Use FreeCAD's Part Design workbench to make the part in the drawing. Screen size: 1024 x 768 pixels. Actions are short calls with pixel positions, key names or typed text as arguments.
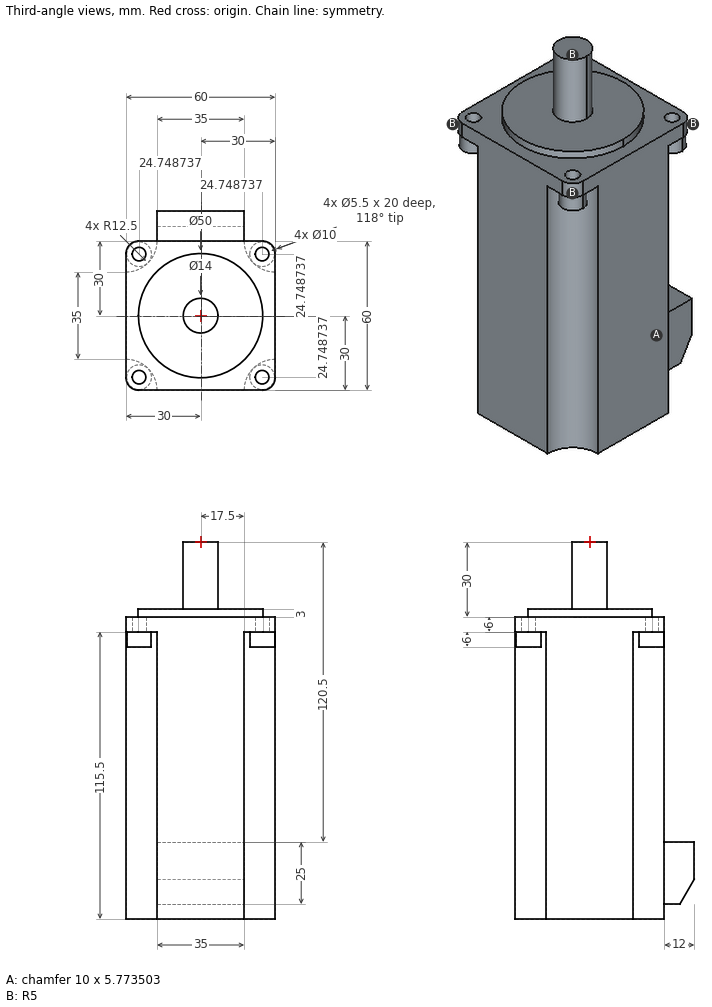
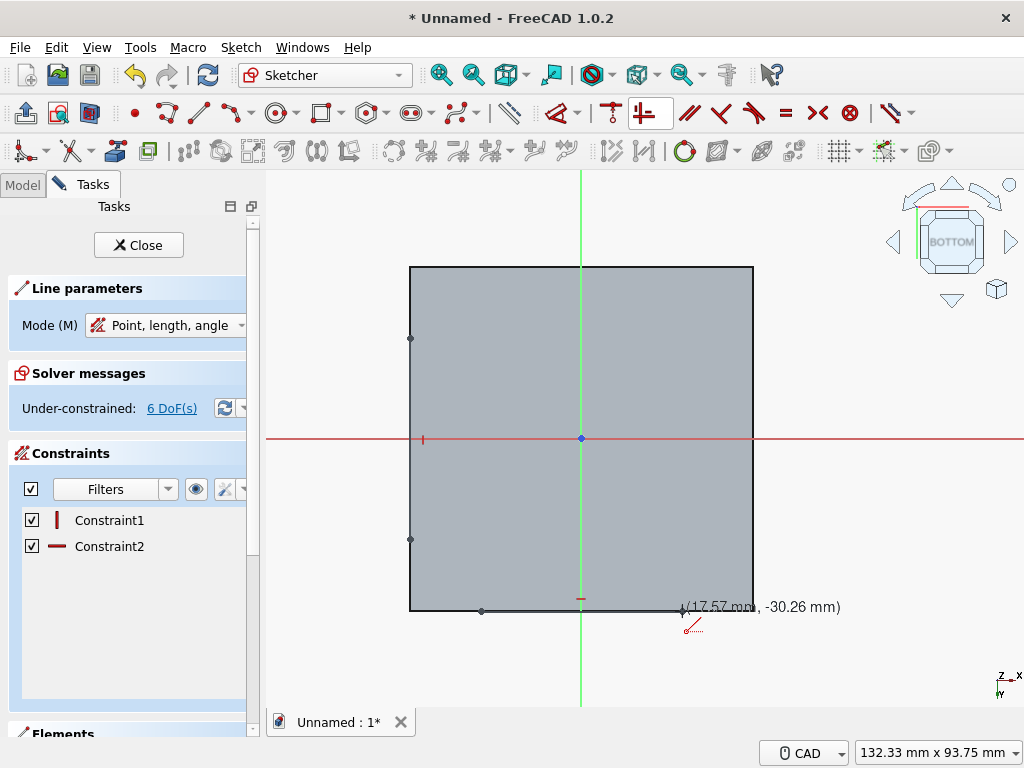
click(753, 539)
click(753, 338)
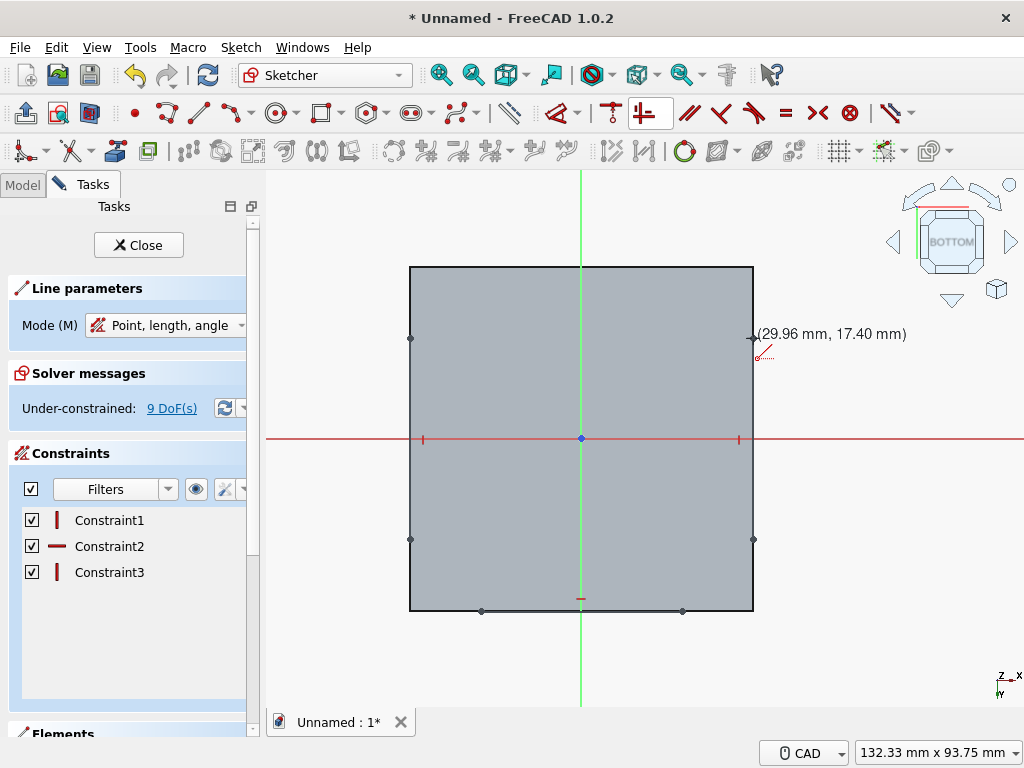
click(682, 267)
click(481, 267)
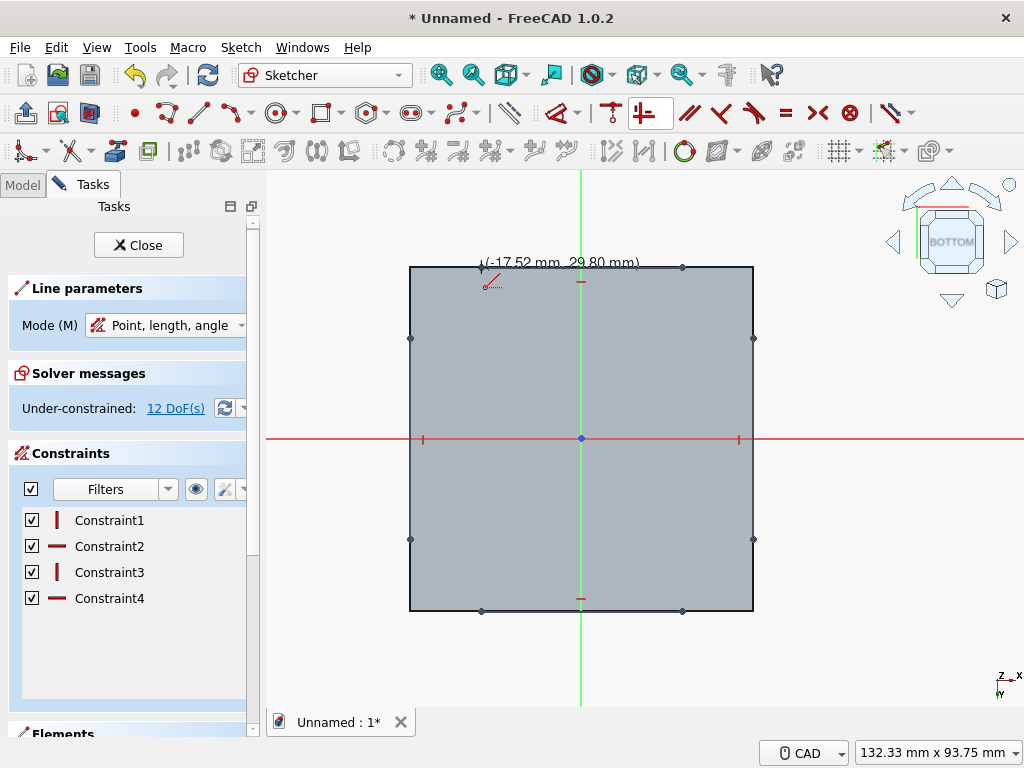
click(232, 114)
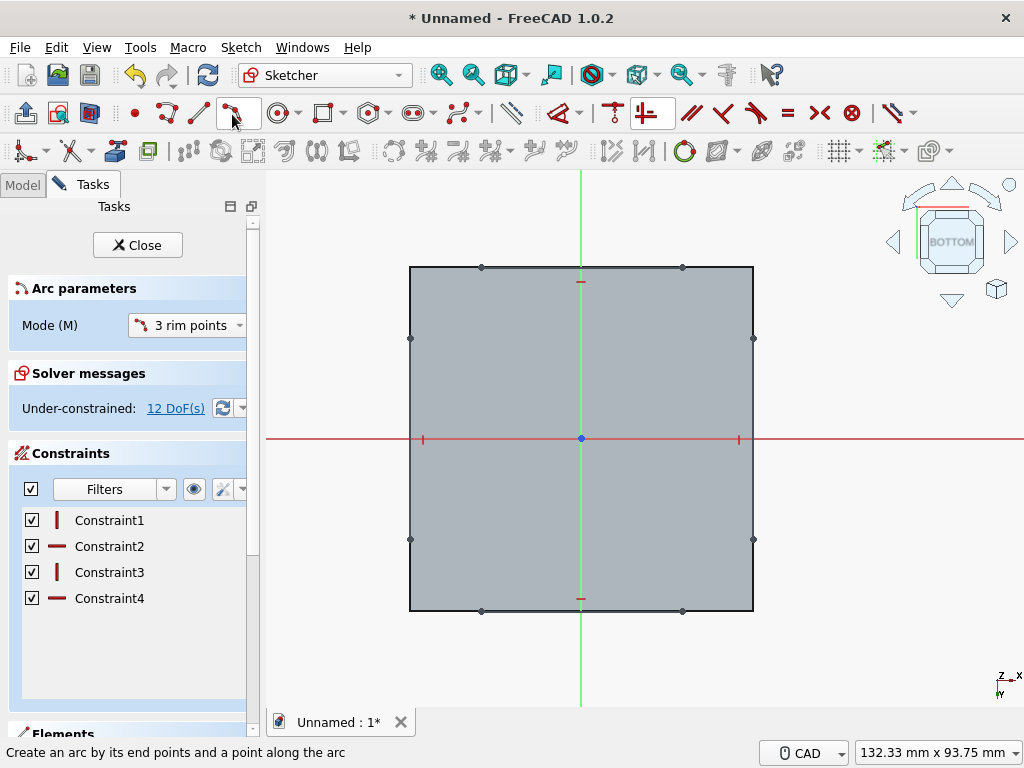
click(410, 540)
click(481, 612)
click(460, 560)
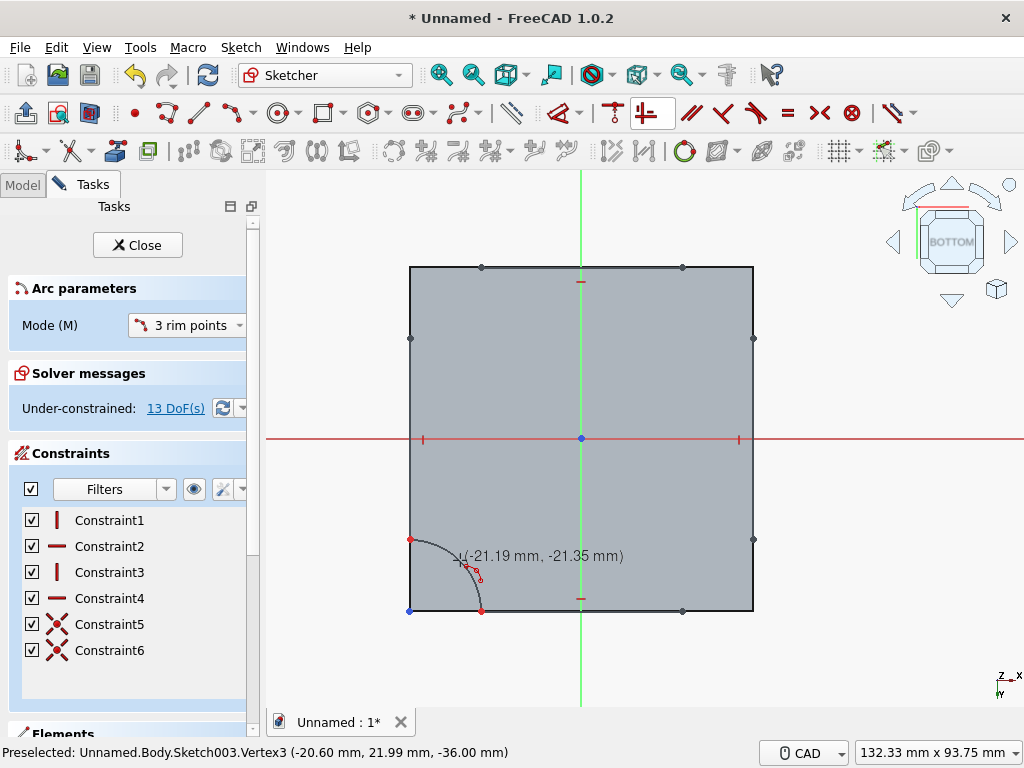
click(682, 612)
click(753, 540)
click(703, 560)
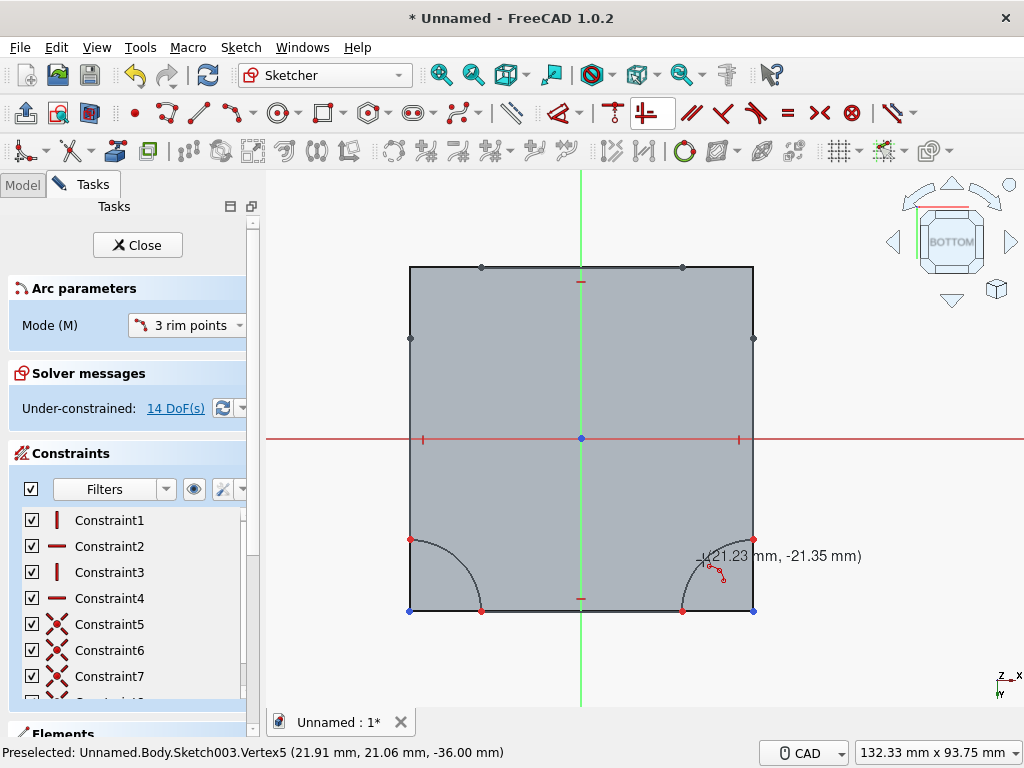
click(753, 339)
click(682, 268)
click(703, 317)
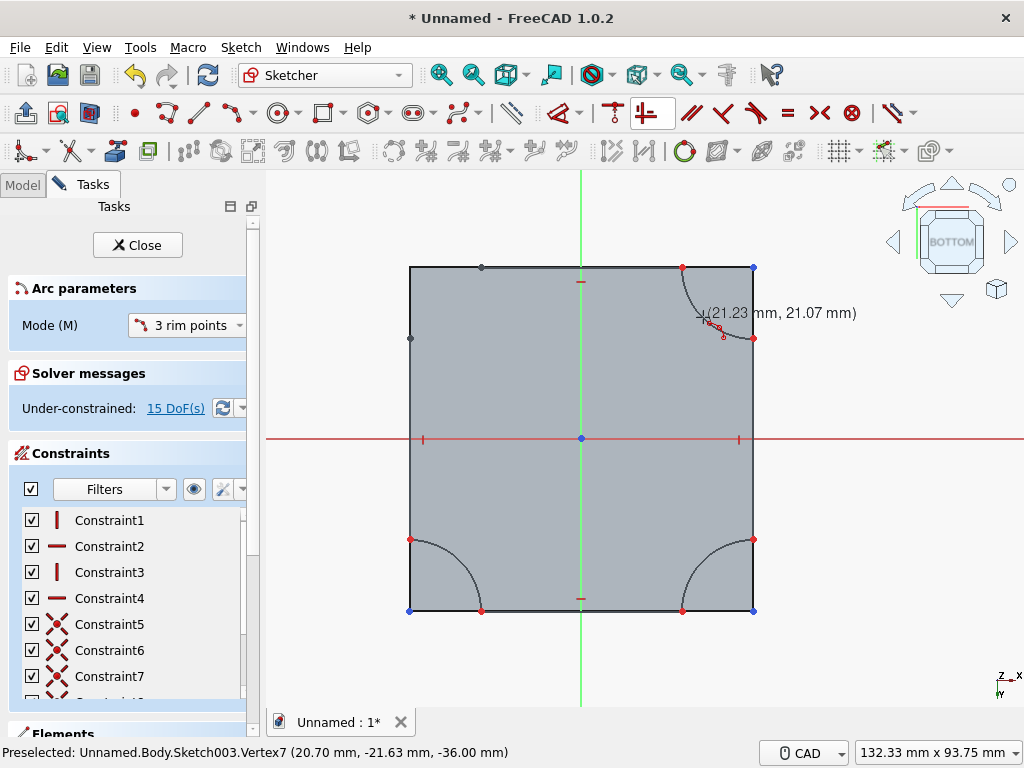
click(481, 268)
click(410, 339)
click(460, 317)
key(Escape)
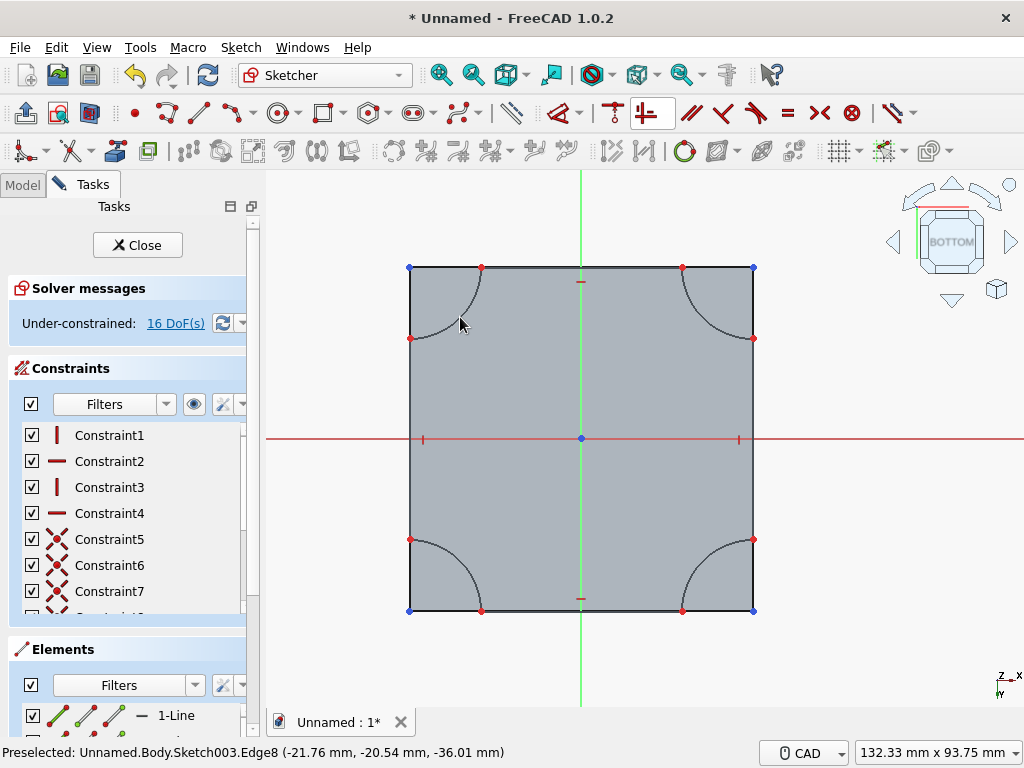
click(473, 580)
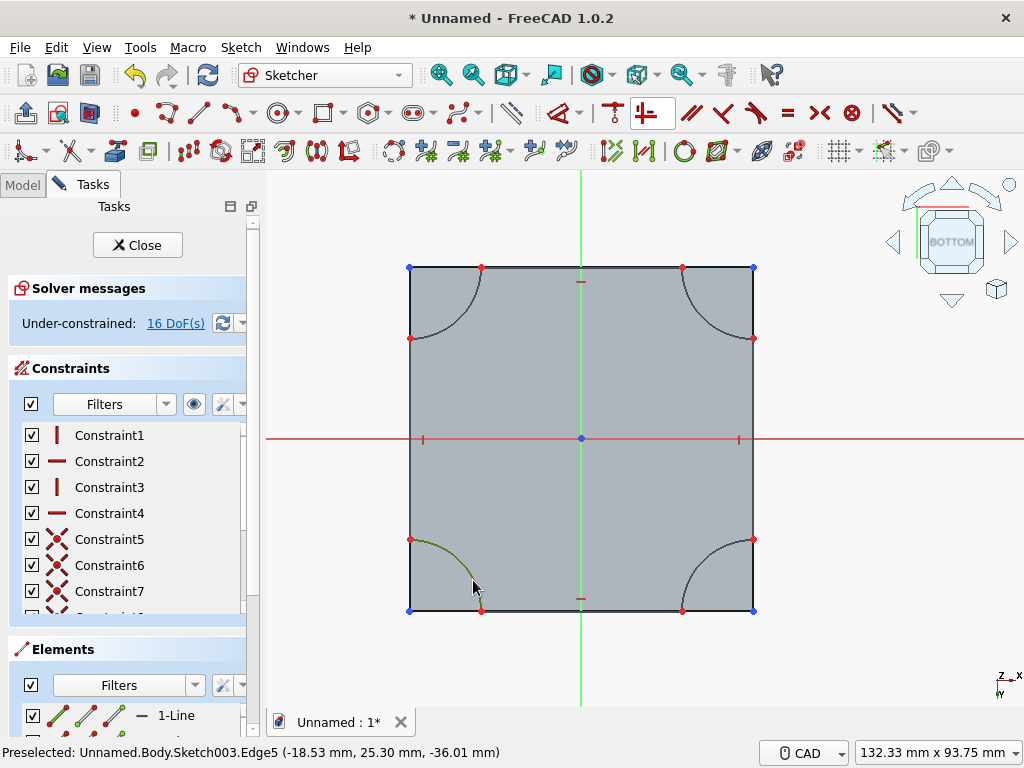
click(721, 548)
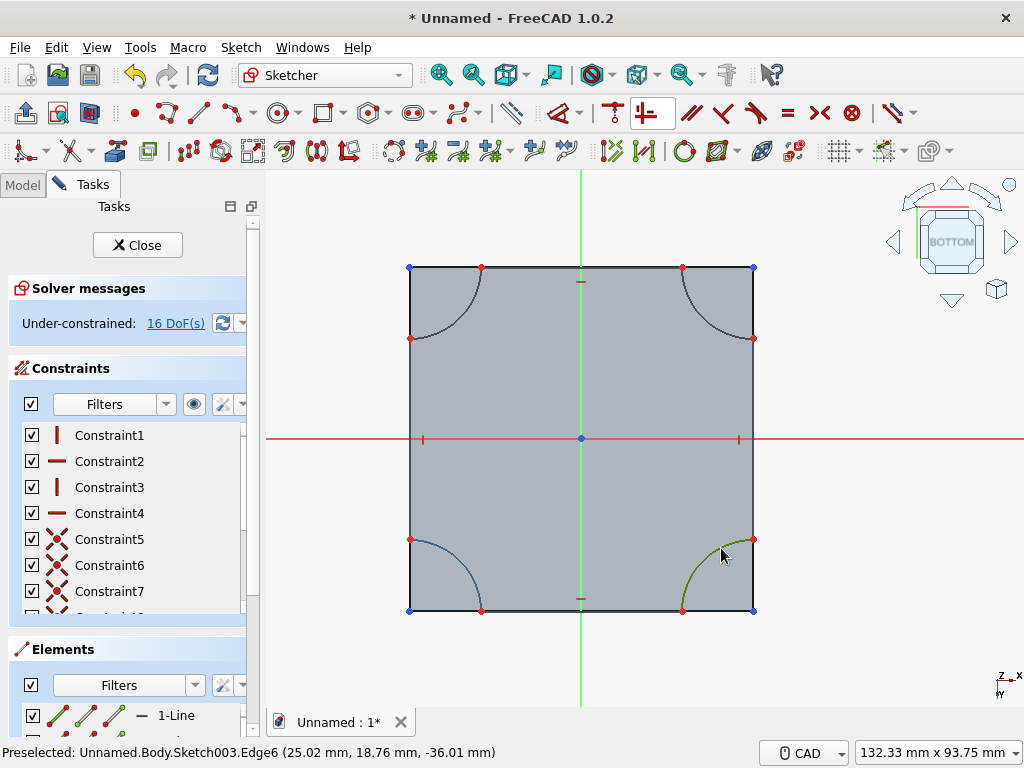
click(690, 300)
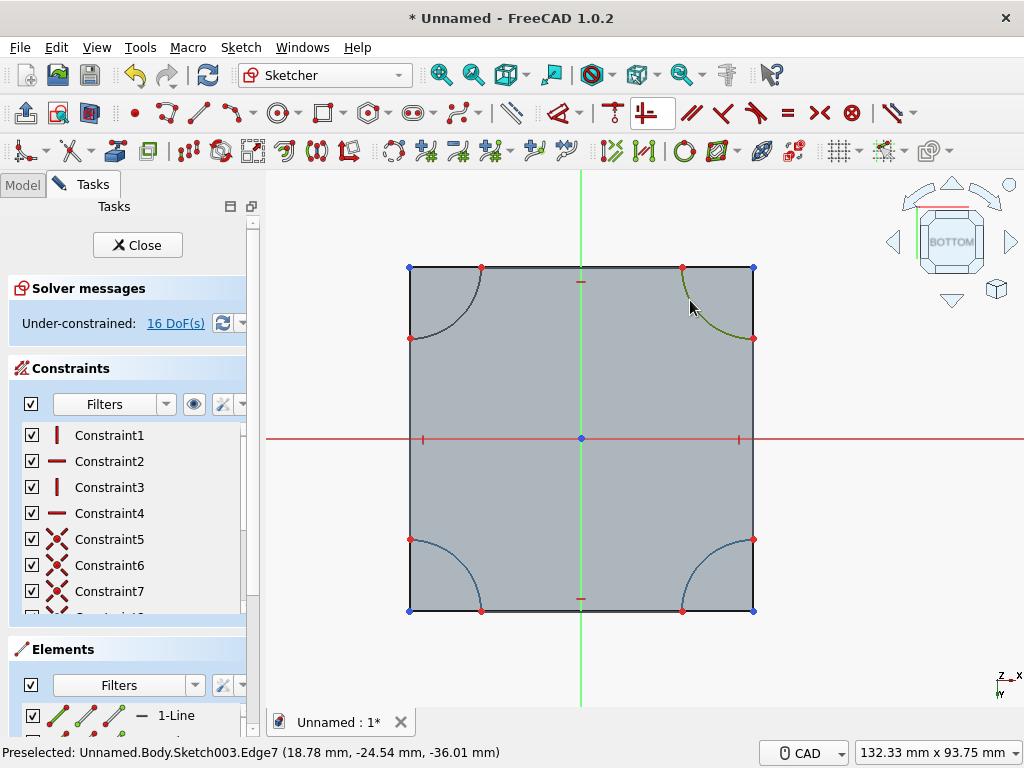
click(442, 331)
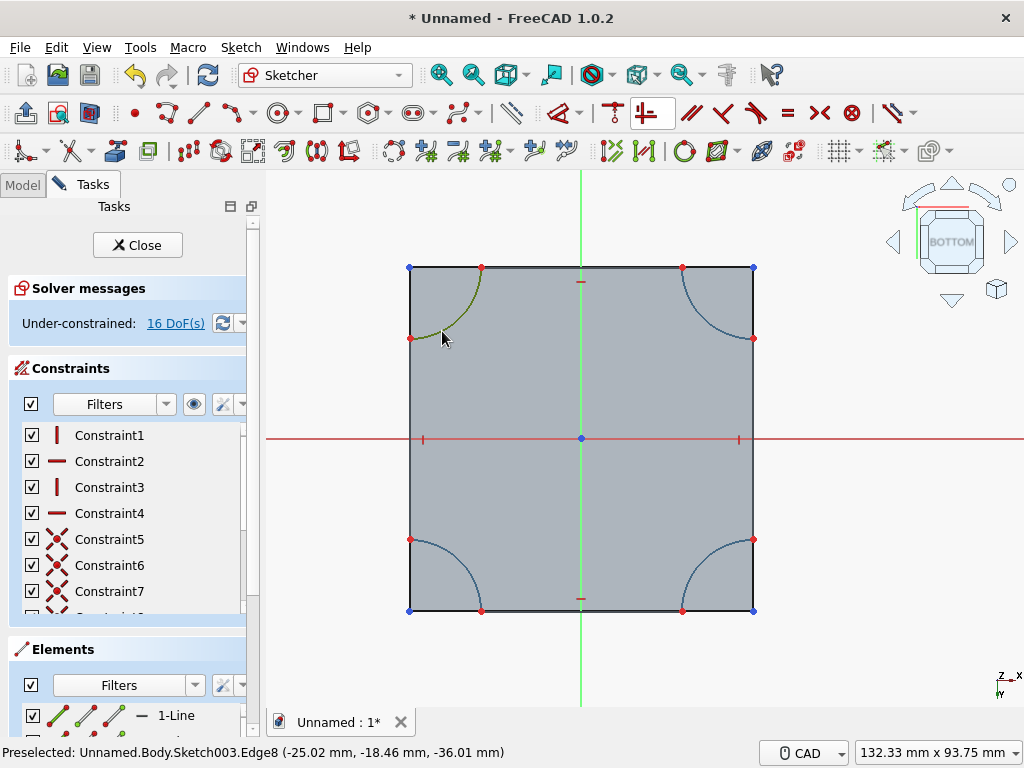
click(788, 114)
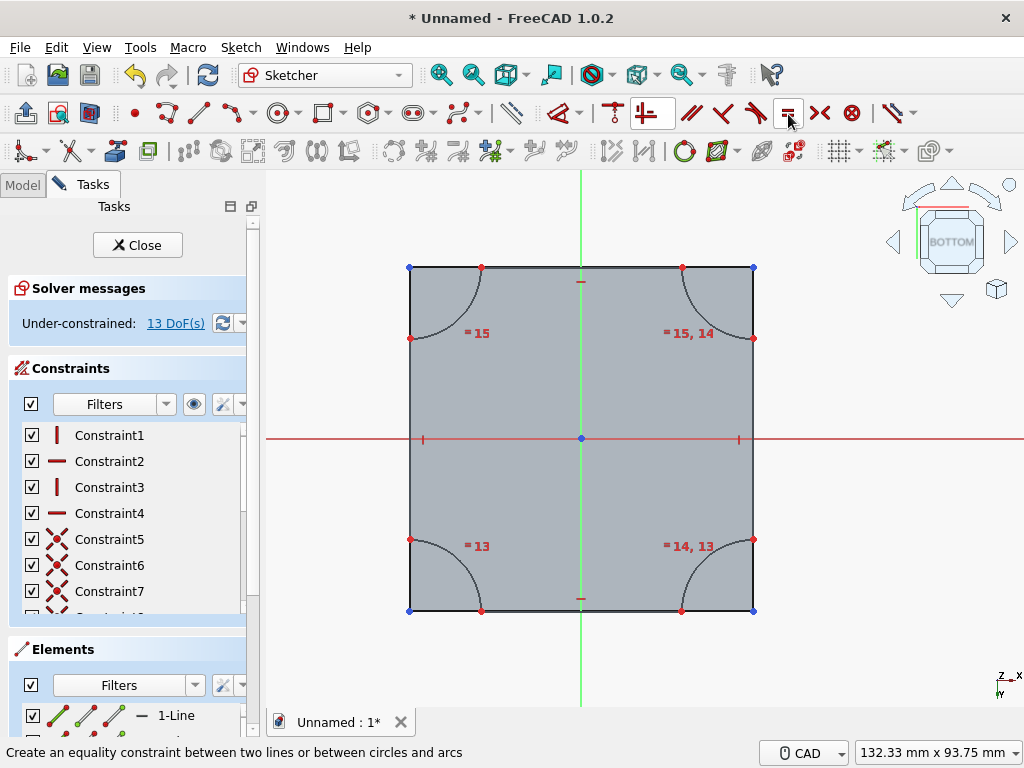
click(409, 612)